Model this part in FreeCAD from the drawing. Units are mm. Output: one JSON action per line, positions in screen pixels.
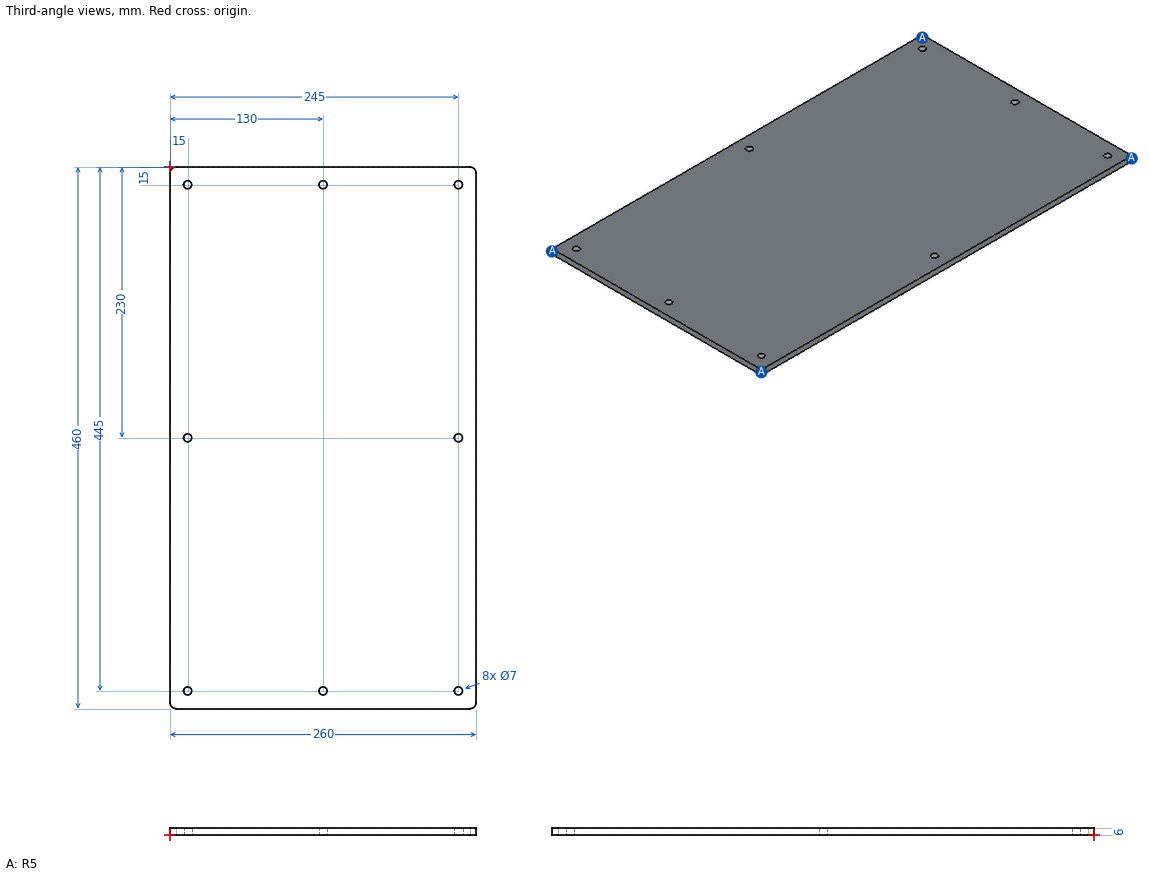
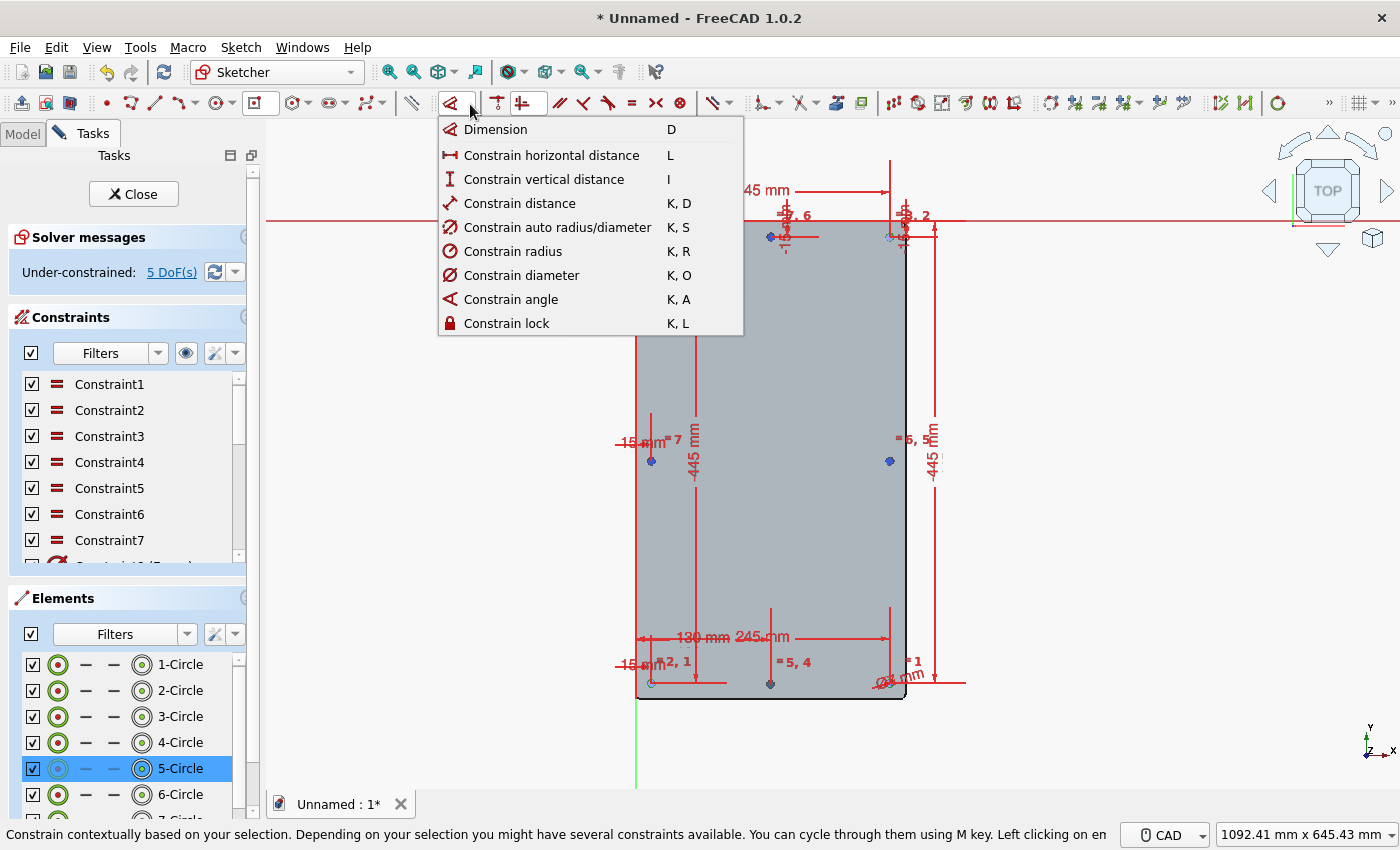
{"action": "left_click", "coordinate": [591, 179]}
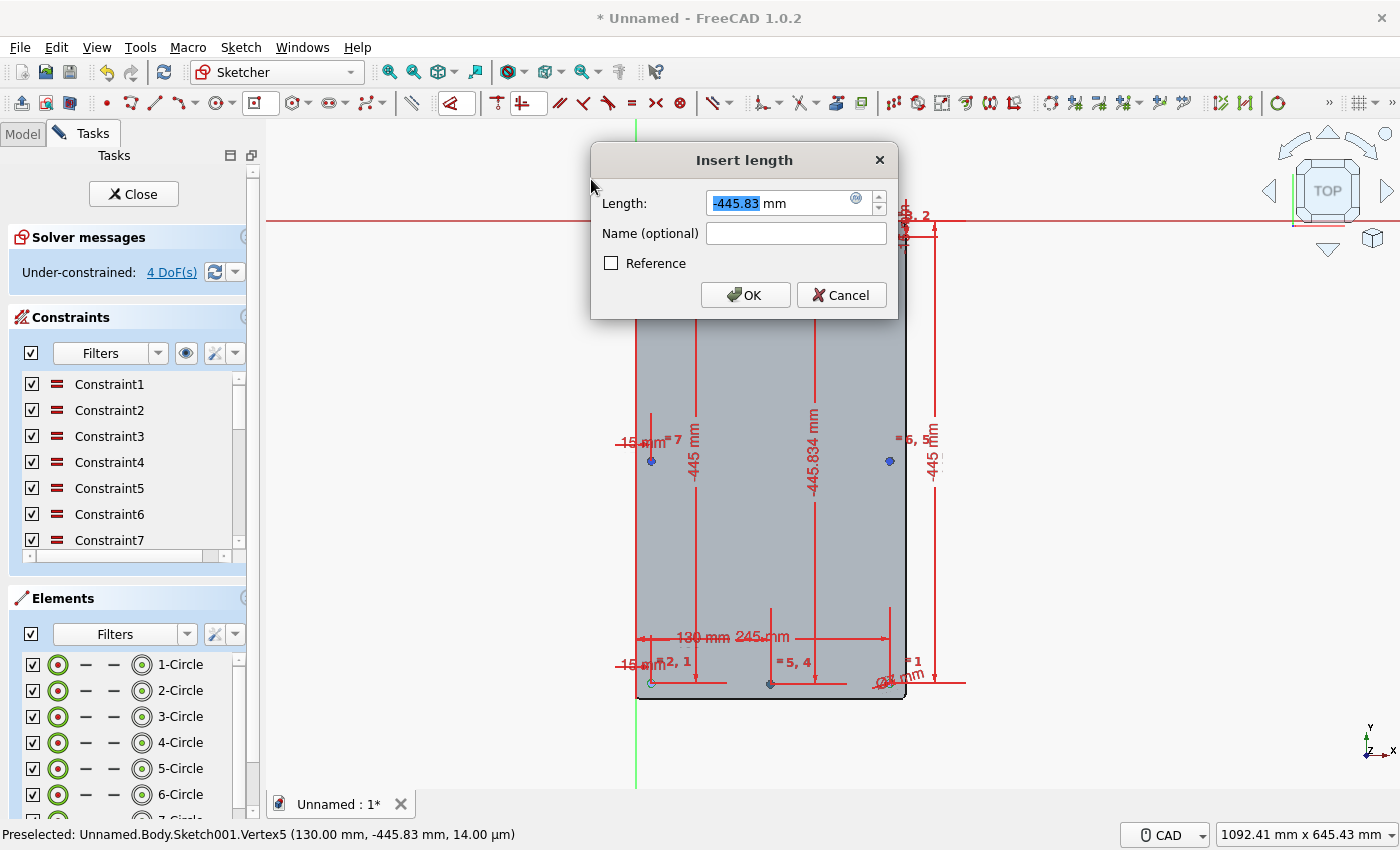
{"action": "type", "text": "-445"}
{"action": "key", "text": "Return"}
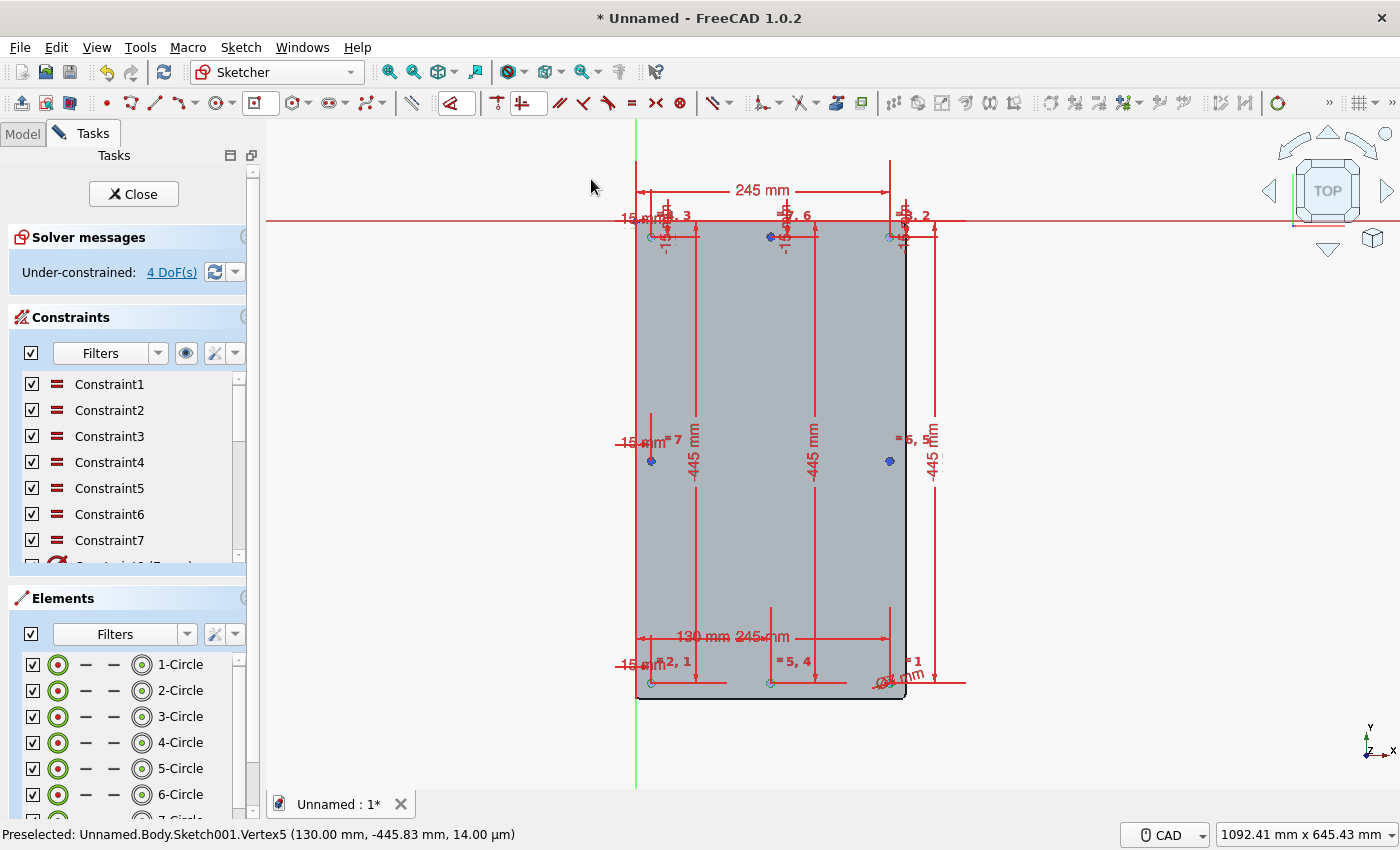
{"action": "left_click", "coordinate": [890, 461]}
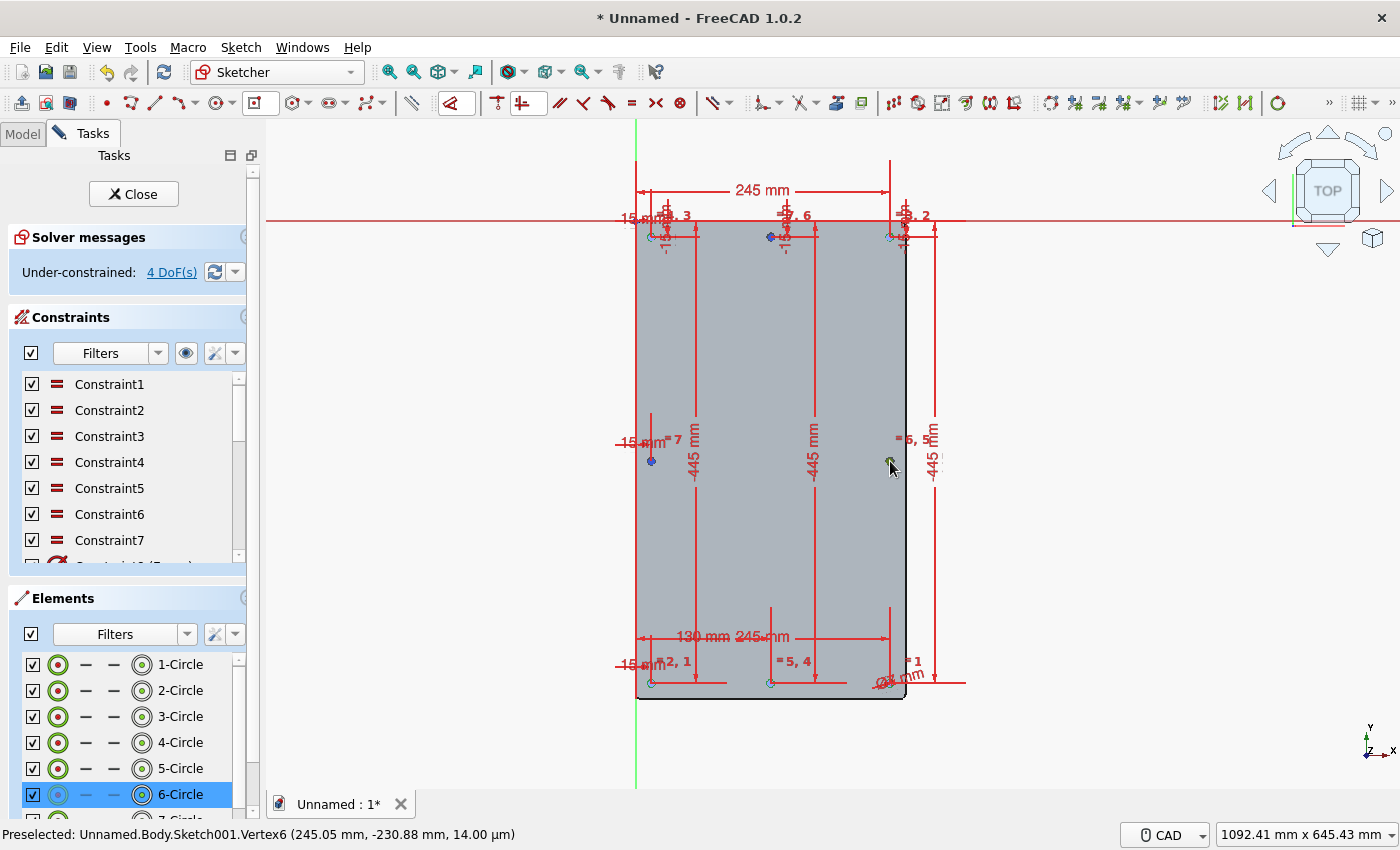
{"action": "key", "text": "l"}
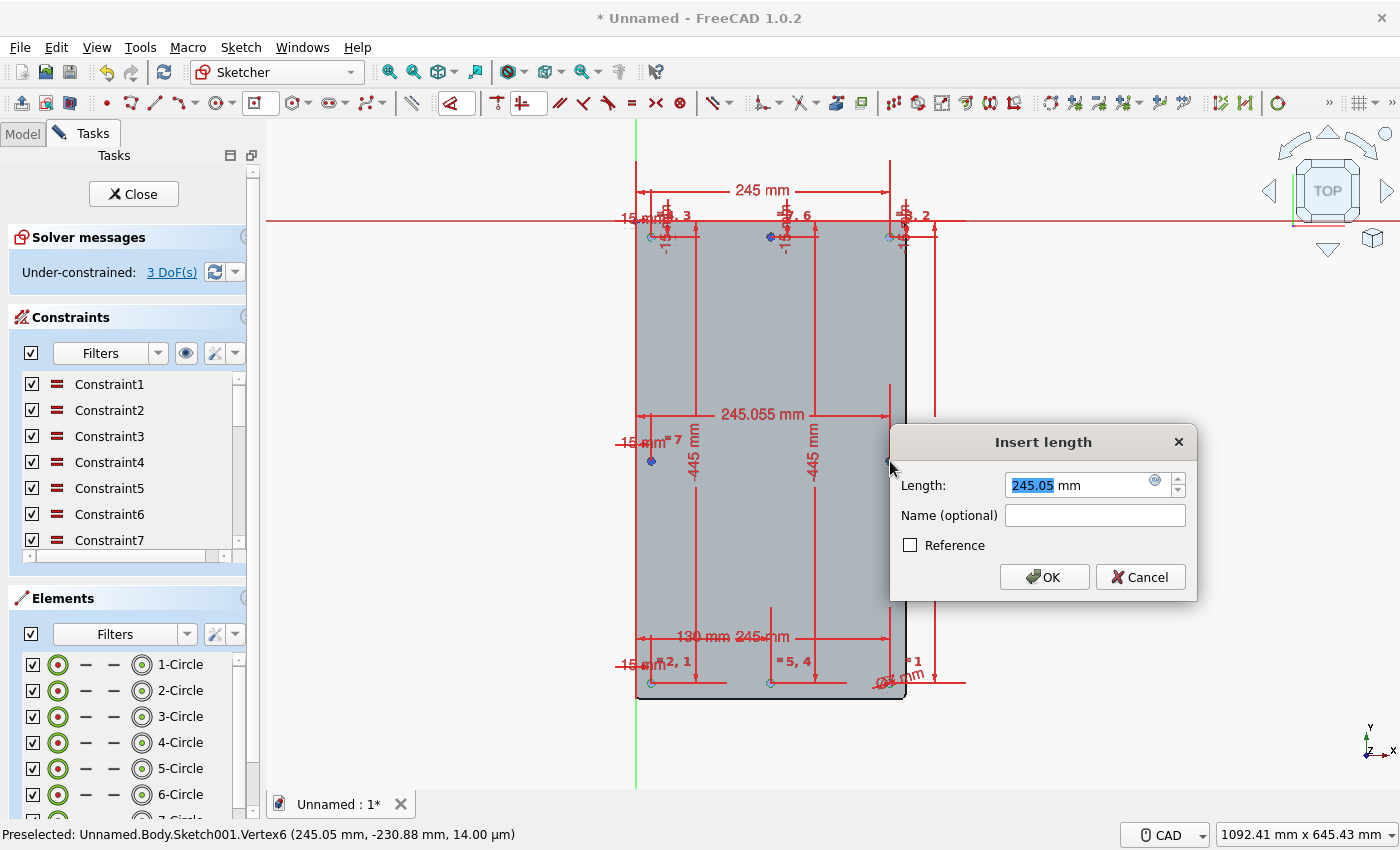
{"action": "type", "text": "245"}
{"action": "key", "text": "Return"}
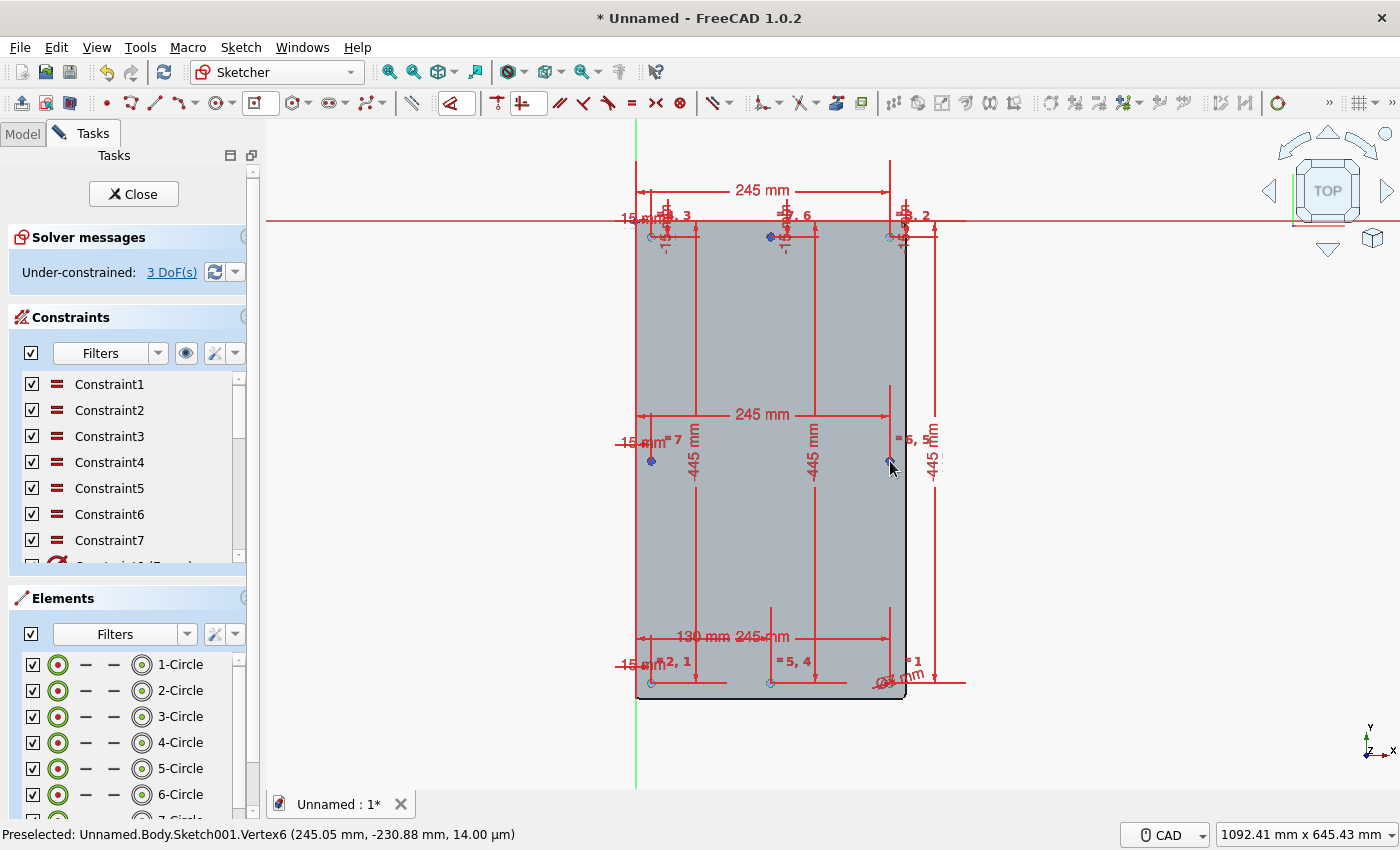
{"action": "left_click", "coordinate": [890, 461]}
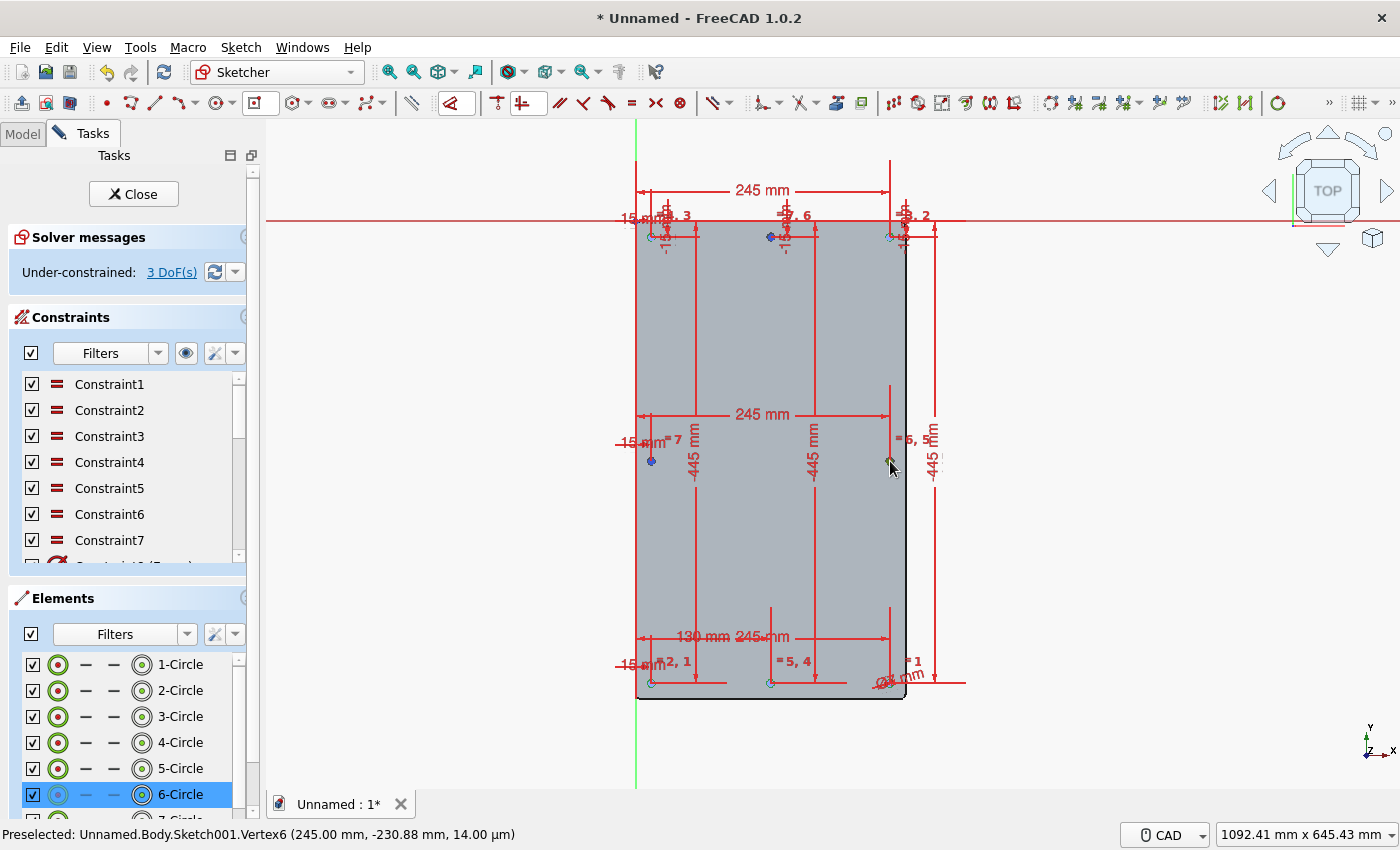
{"action": "key", "text": "i"}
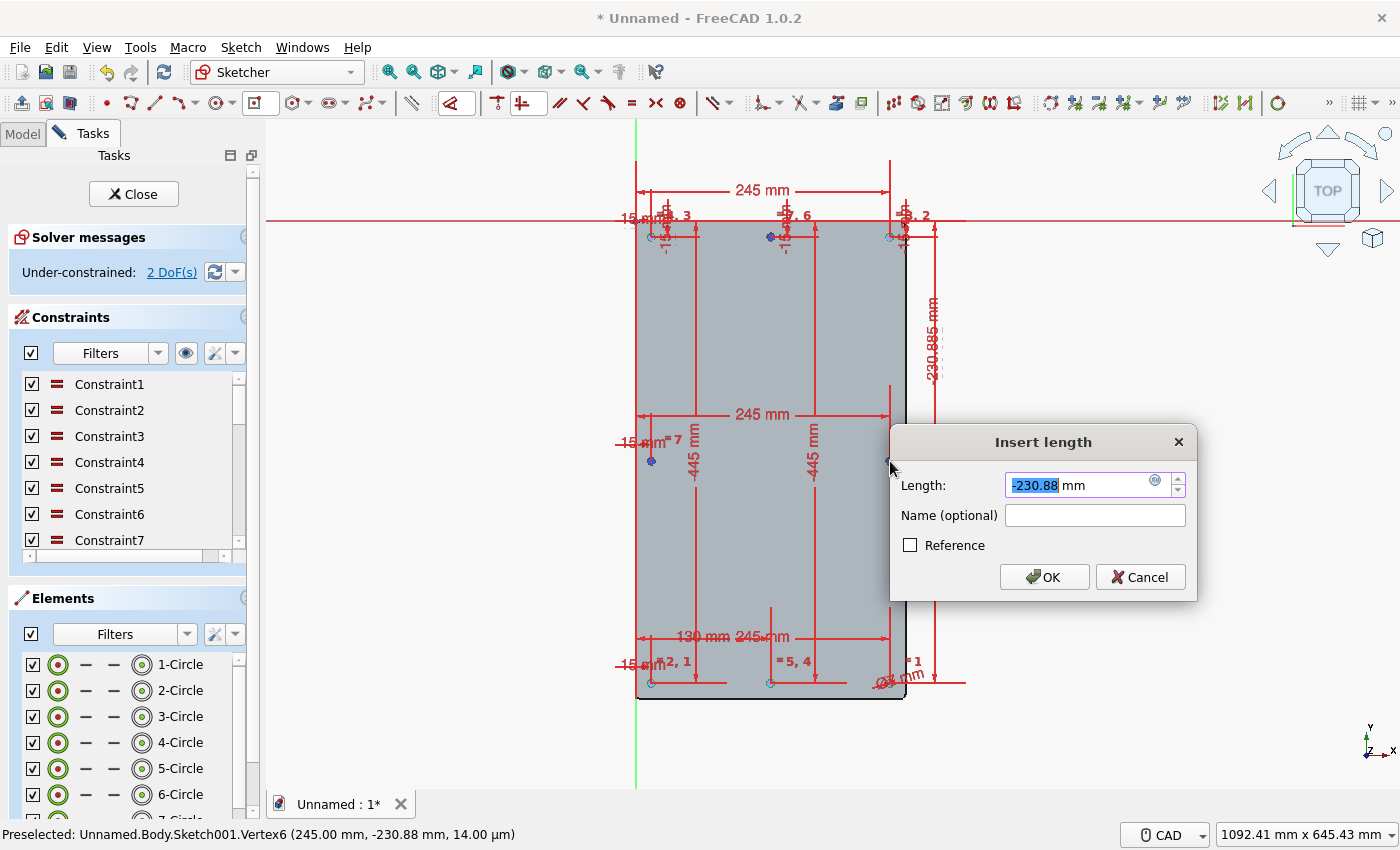
{"action": "type", "text": "-230"}
{"action": "key", "text": "Return"}